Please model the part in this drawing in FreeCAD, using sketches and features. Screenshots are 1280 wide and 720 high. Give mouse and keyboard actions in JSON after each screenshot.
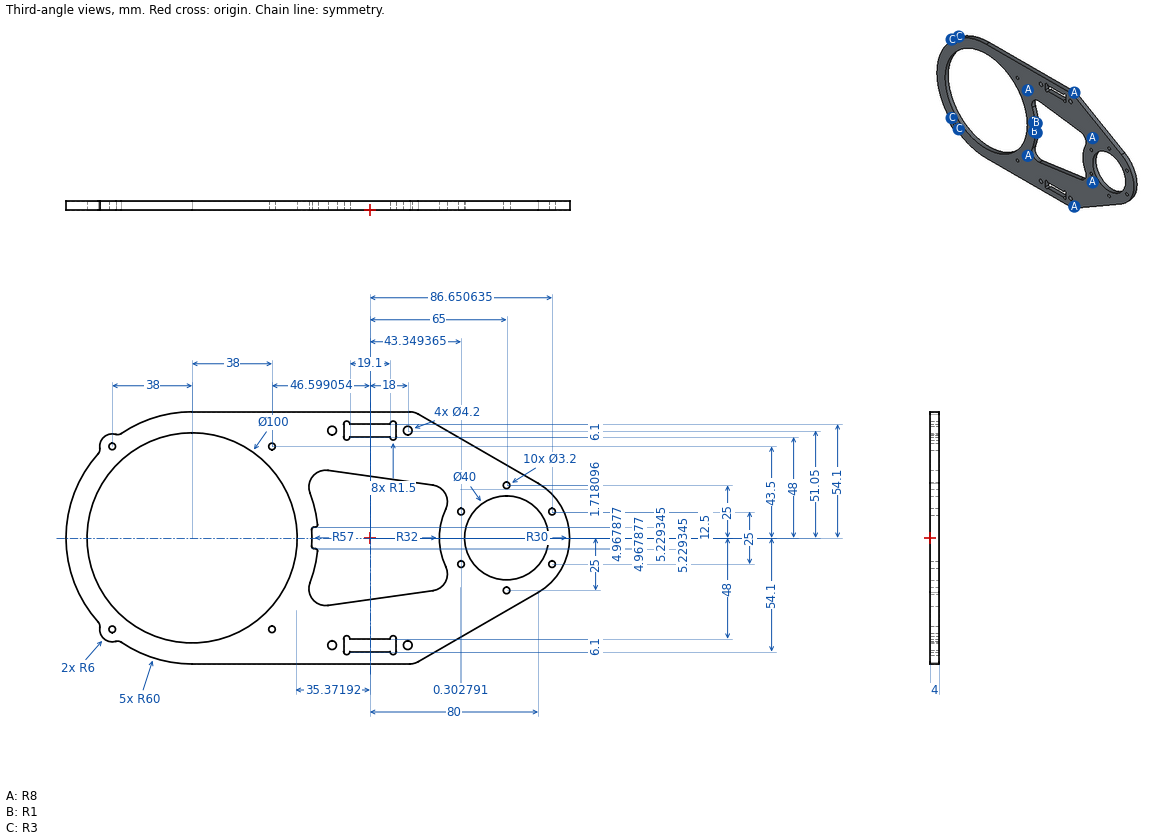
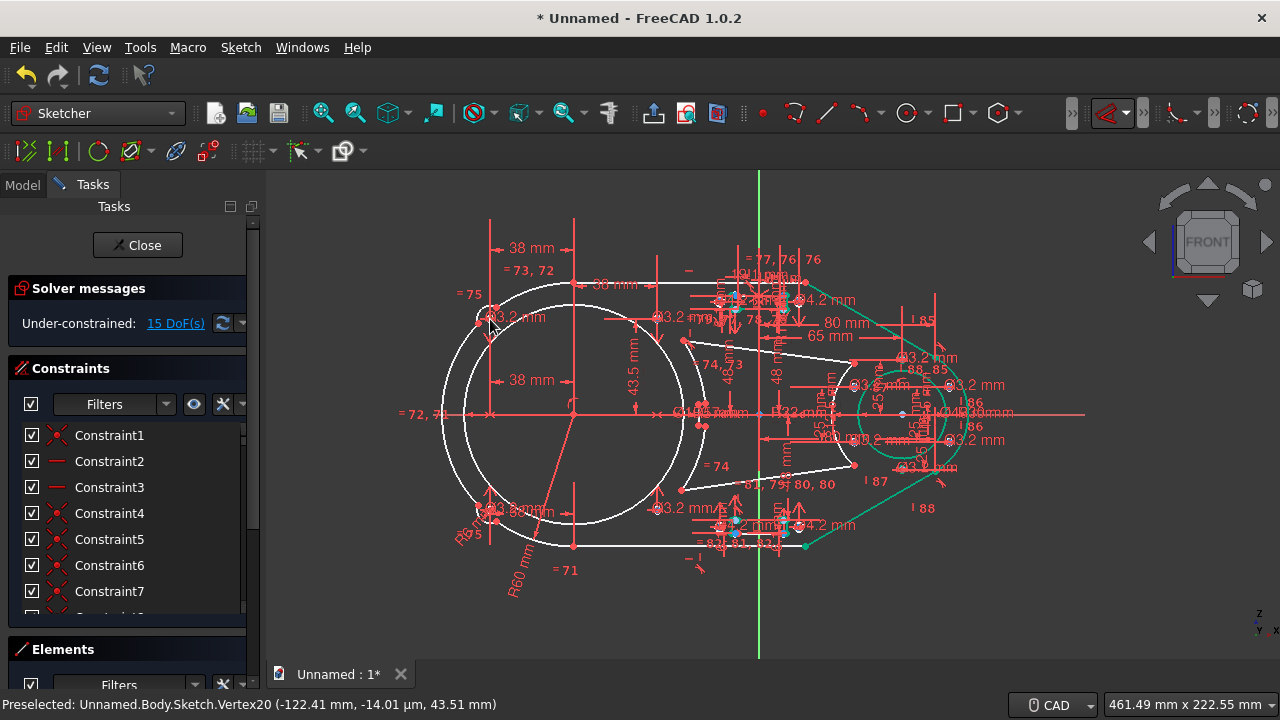
{"action": "left_click", "coordinate": [1128, 114]}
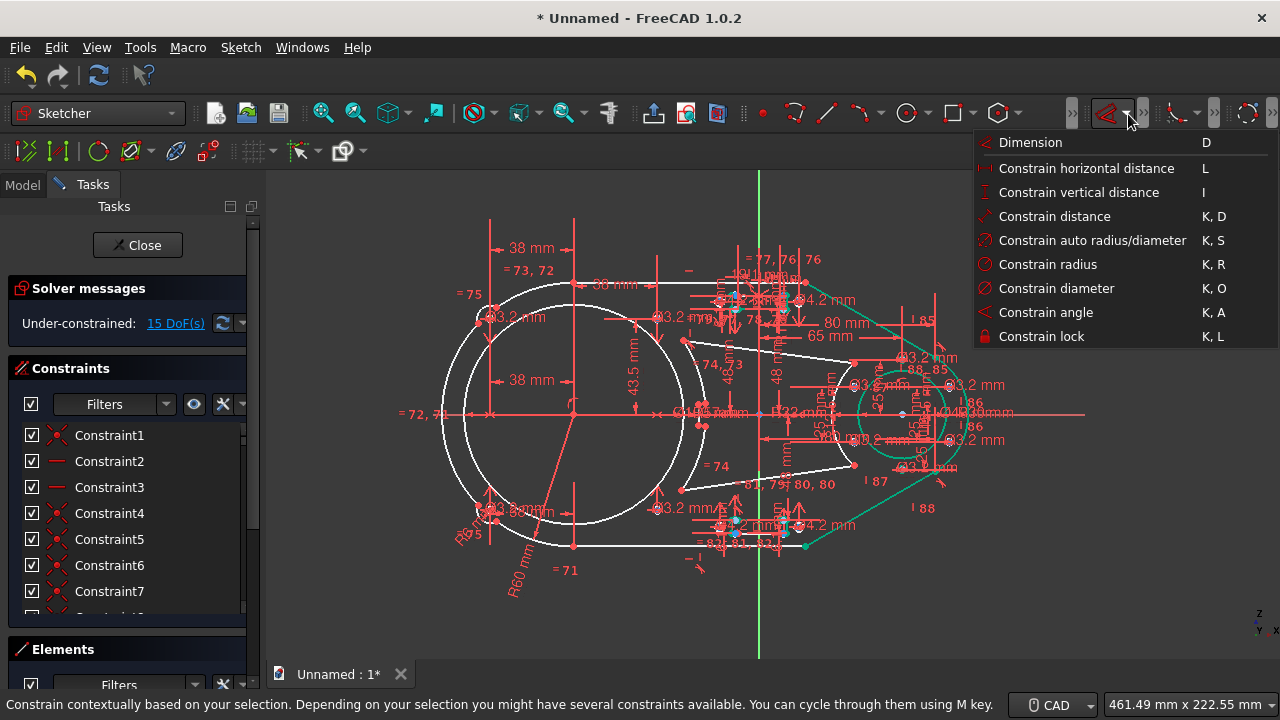
{"action": "left_click", "coordinate": [1126, 192]}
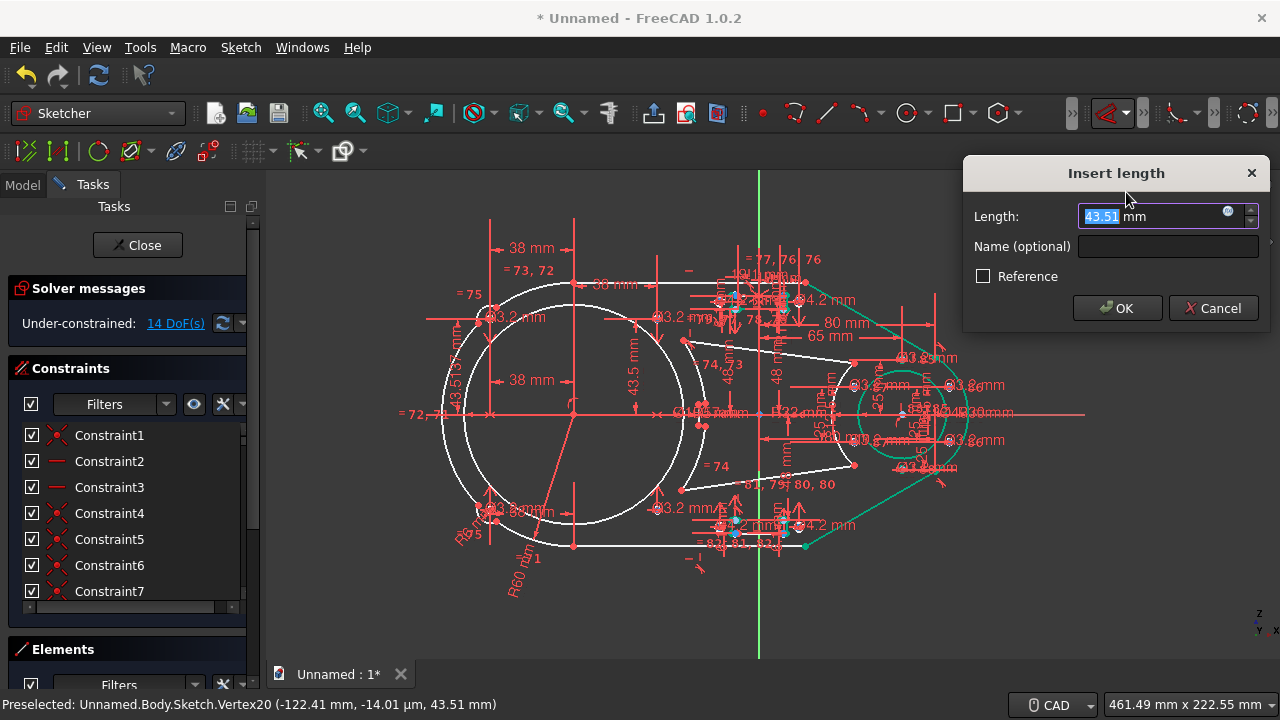
{"action": "type", "text": "43.5"}
{"action": "key", "text": "Return"}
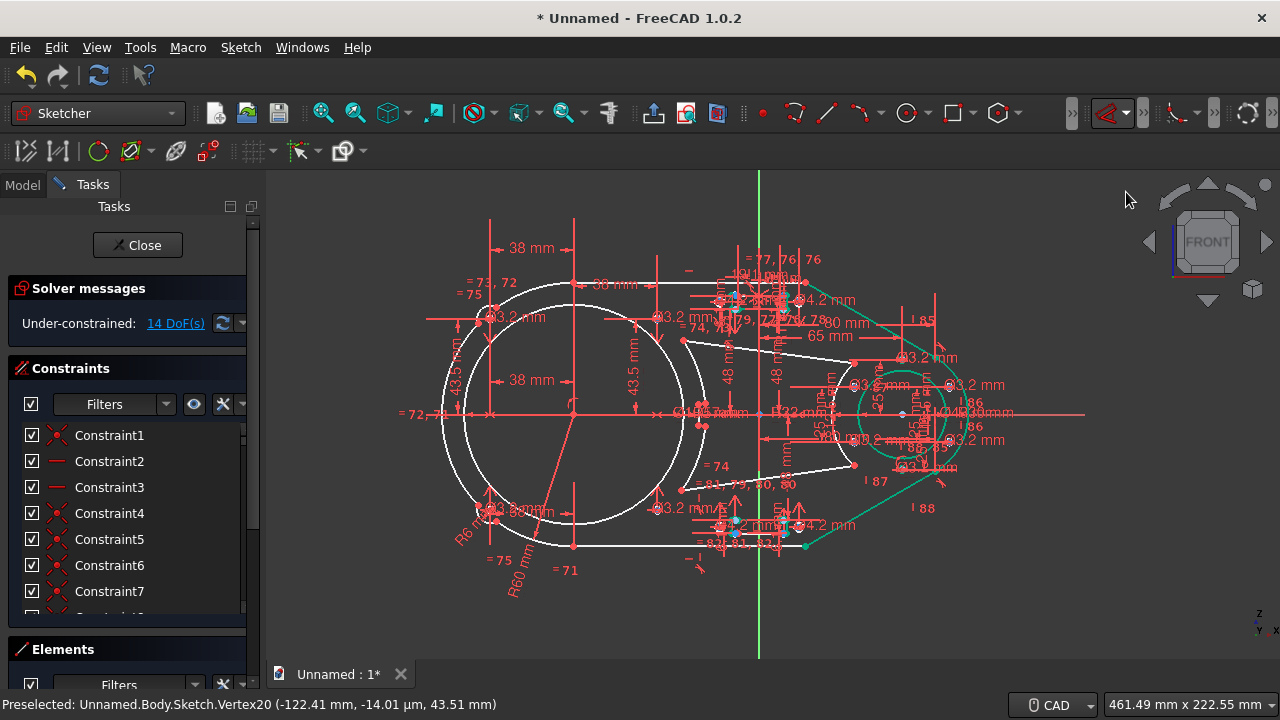
{"action": "scroll", "coordinate": [780, 296], "scroll_direction": "up", "scroll_amount": 7}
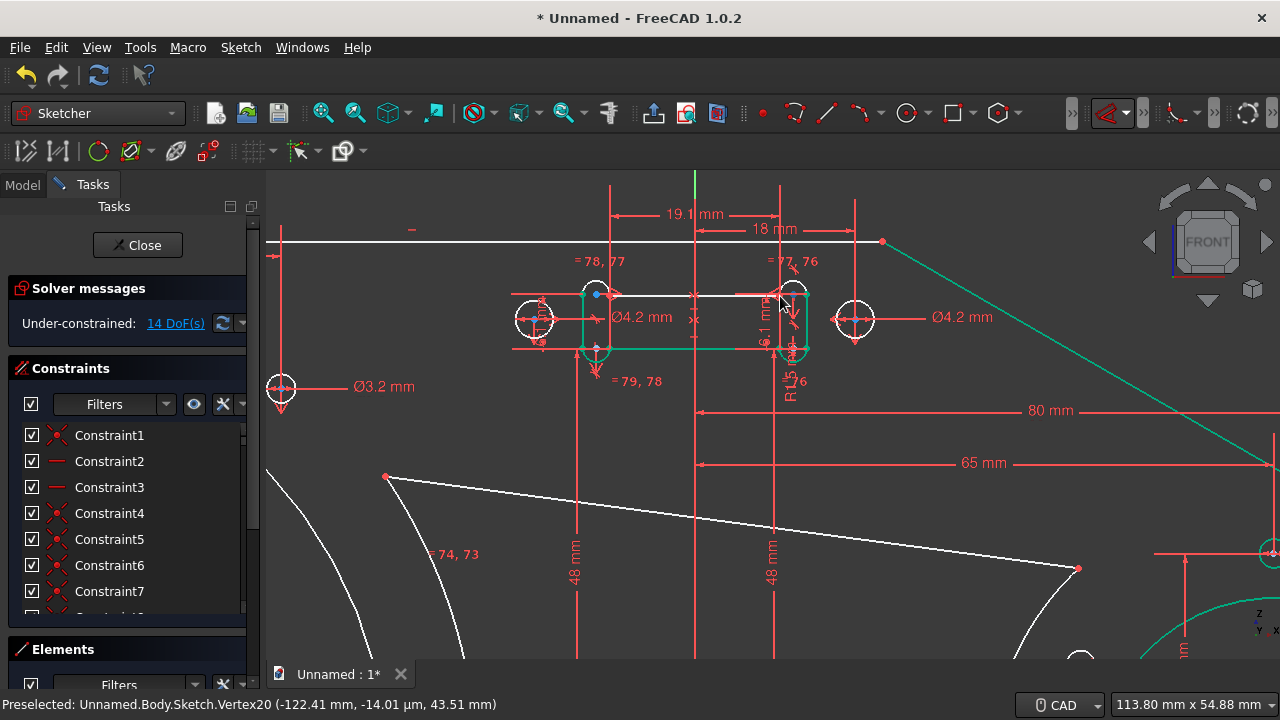
{"action": "left_click", "coordinate": [780, 296]}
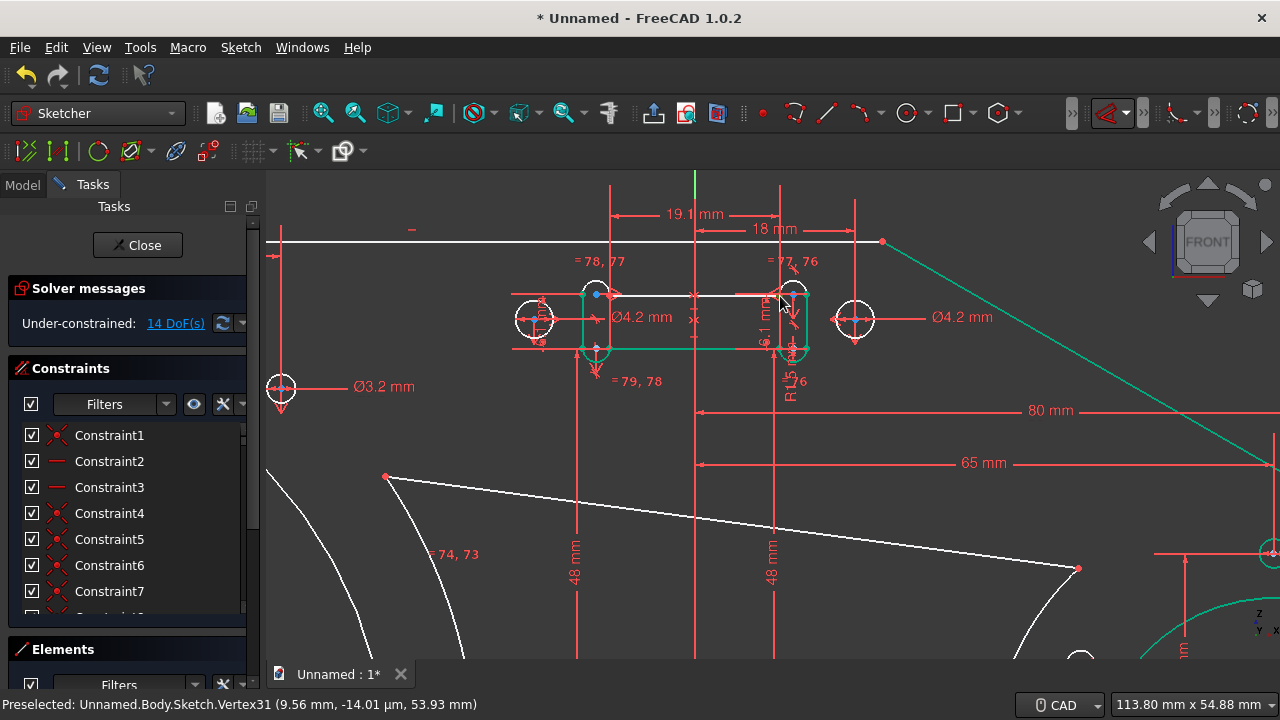
{"action": "key", "text": "i"}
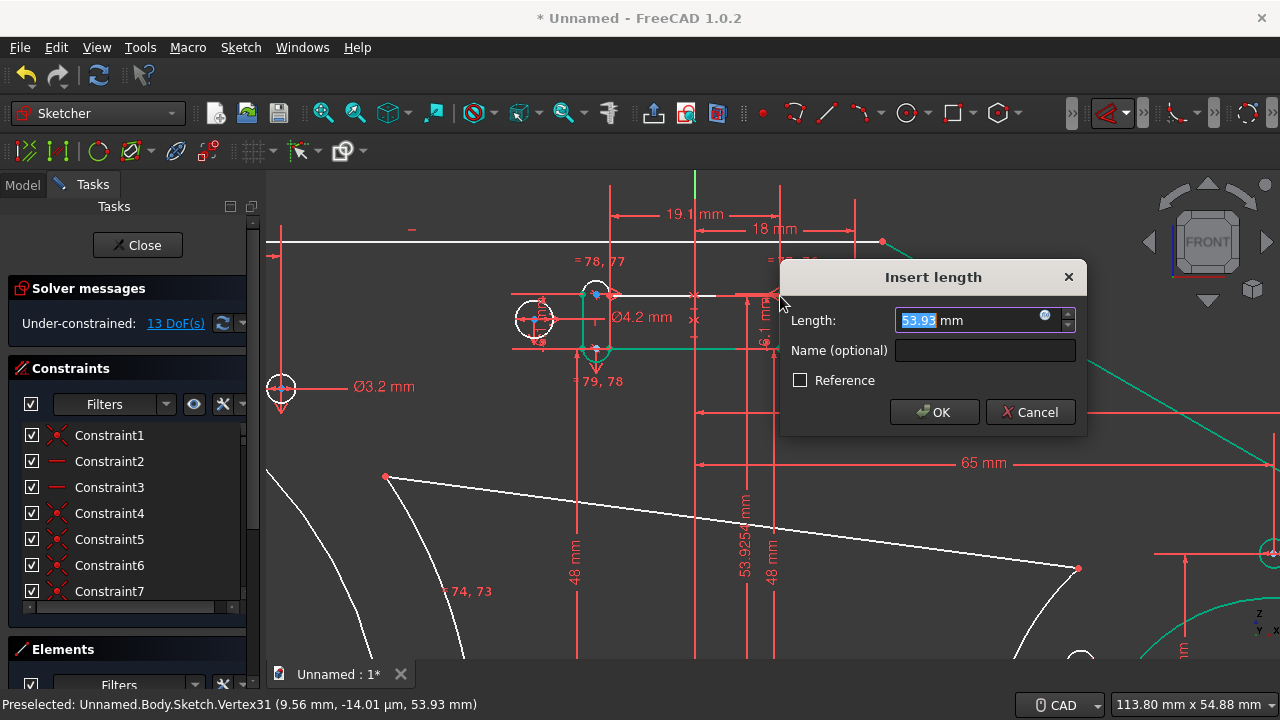
{"action": "type", "text": "54.1"}
{"action": "key", "text": "Return"}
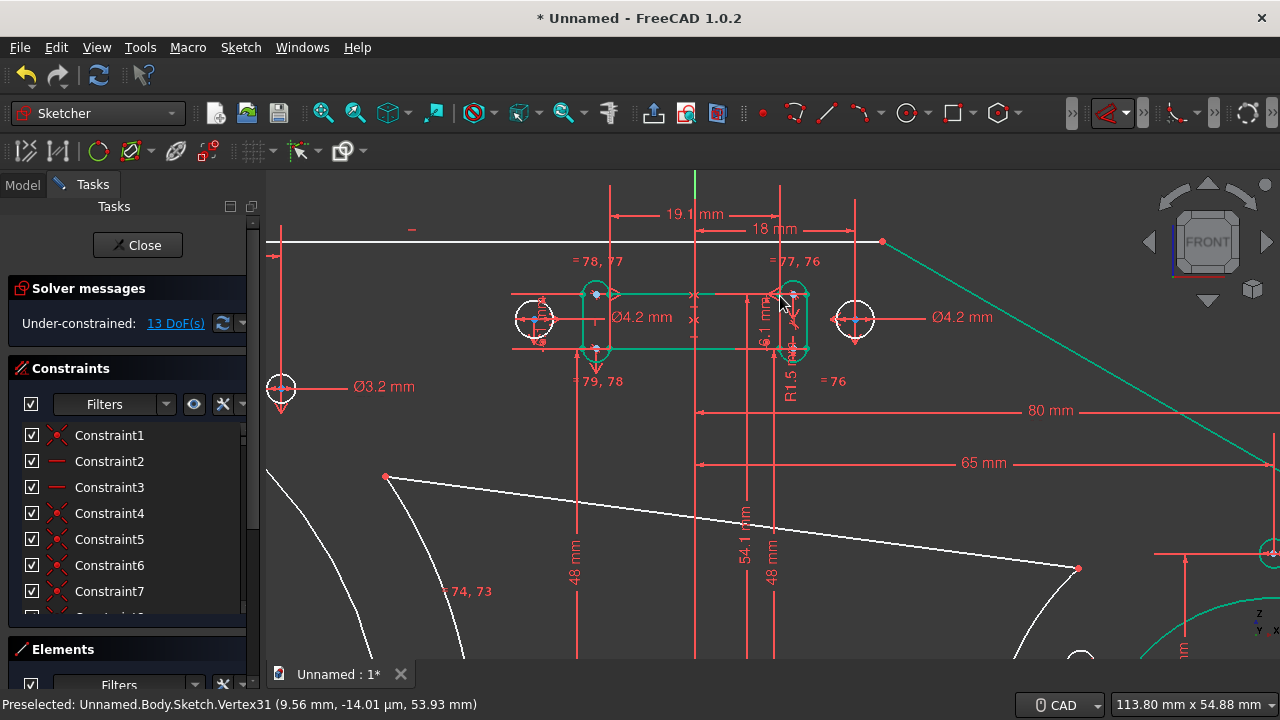
{"action": "scroll", "coordinate": [780, 296], "scroll_direction": "down", "scroll_amount": 7}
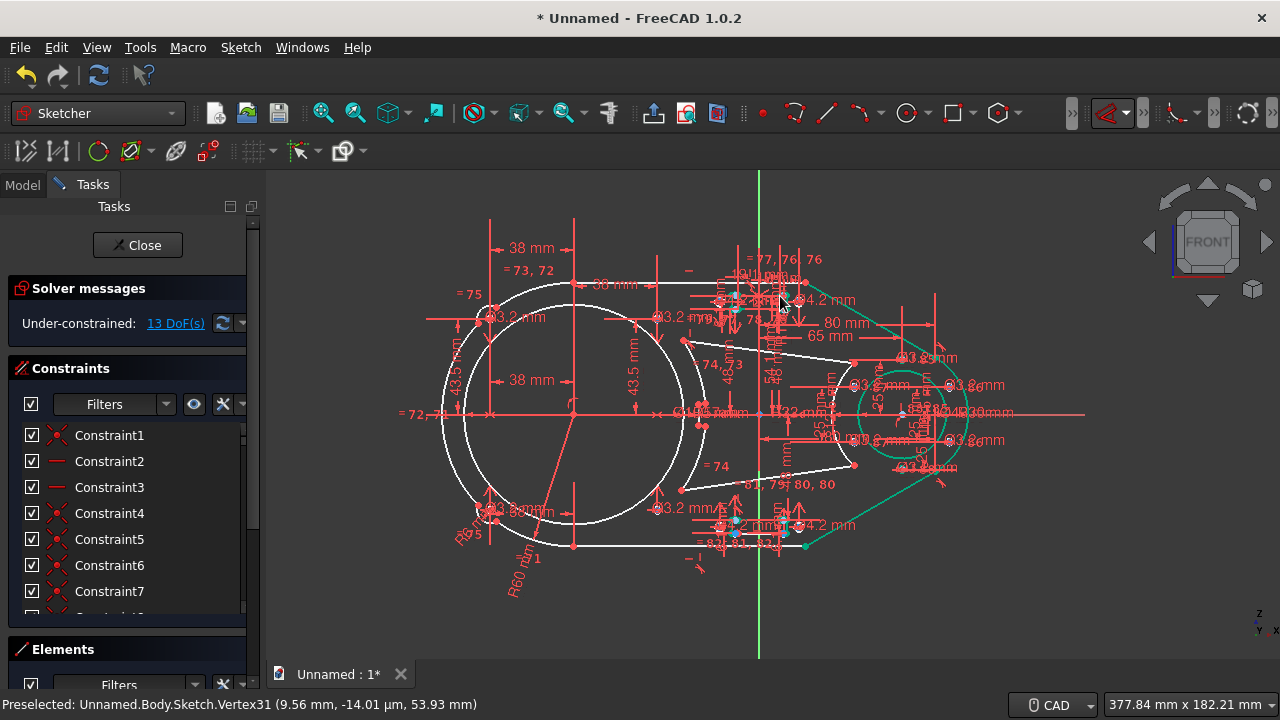
{"action": "scroll", "coordinate": [738, 534], "scroll_direction": "up", "scroll_amount": 7}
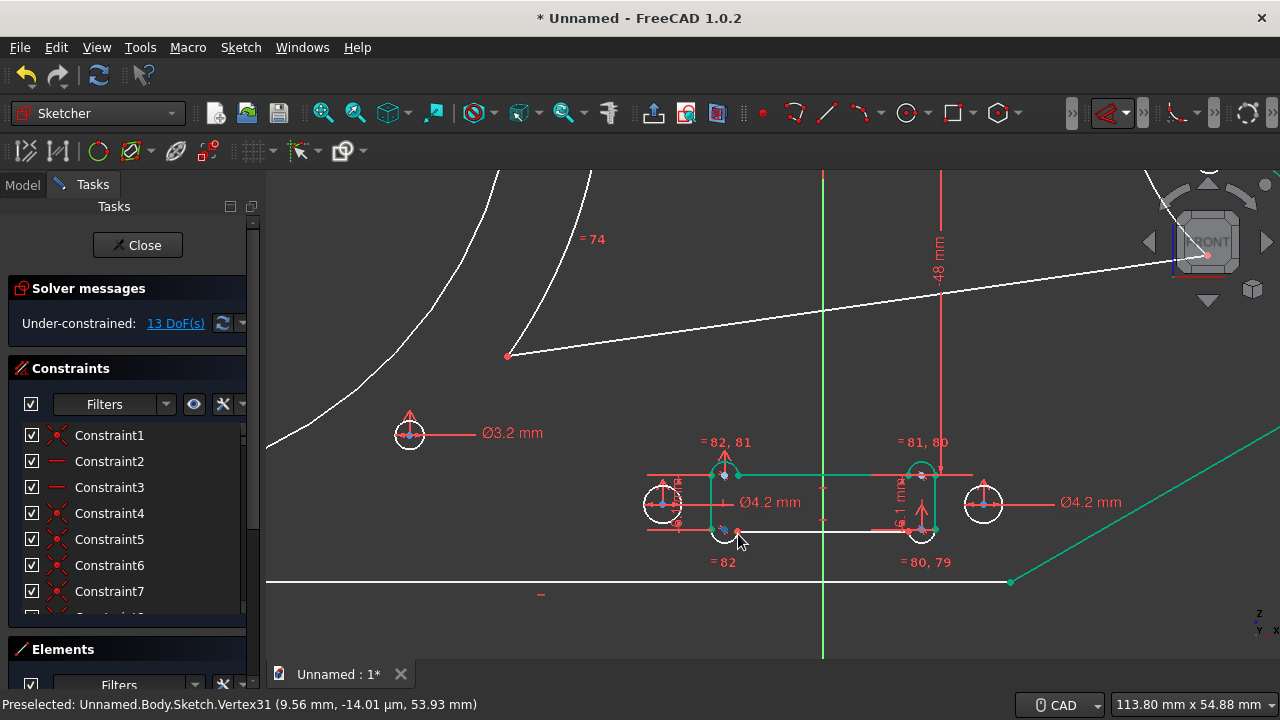
{"action": "left_click", "coordinate": [738, 532]}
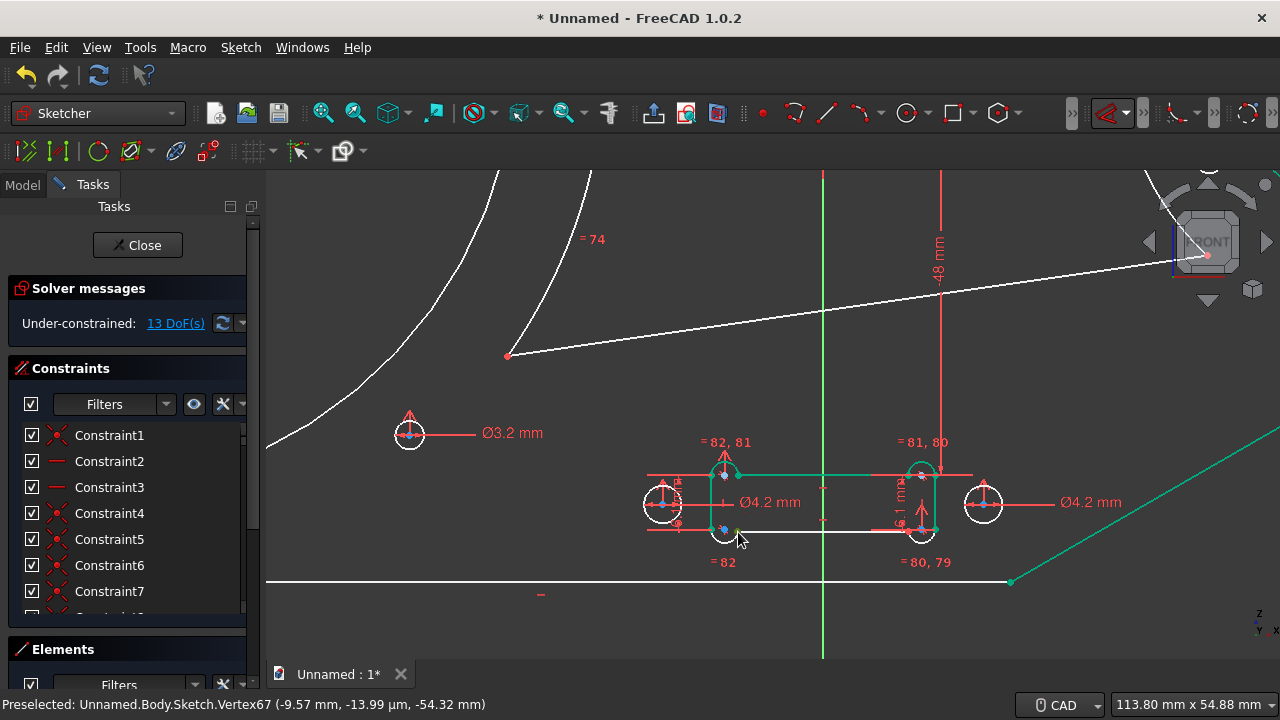
{"action": "left_click", "coordinate": [1128, 114]}